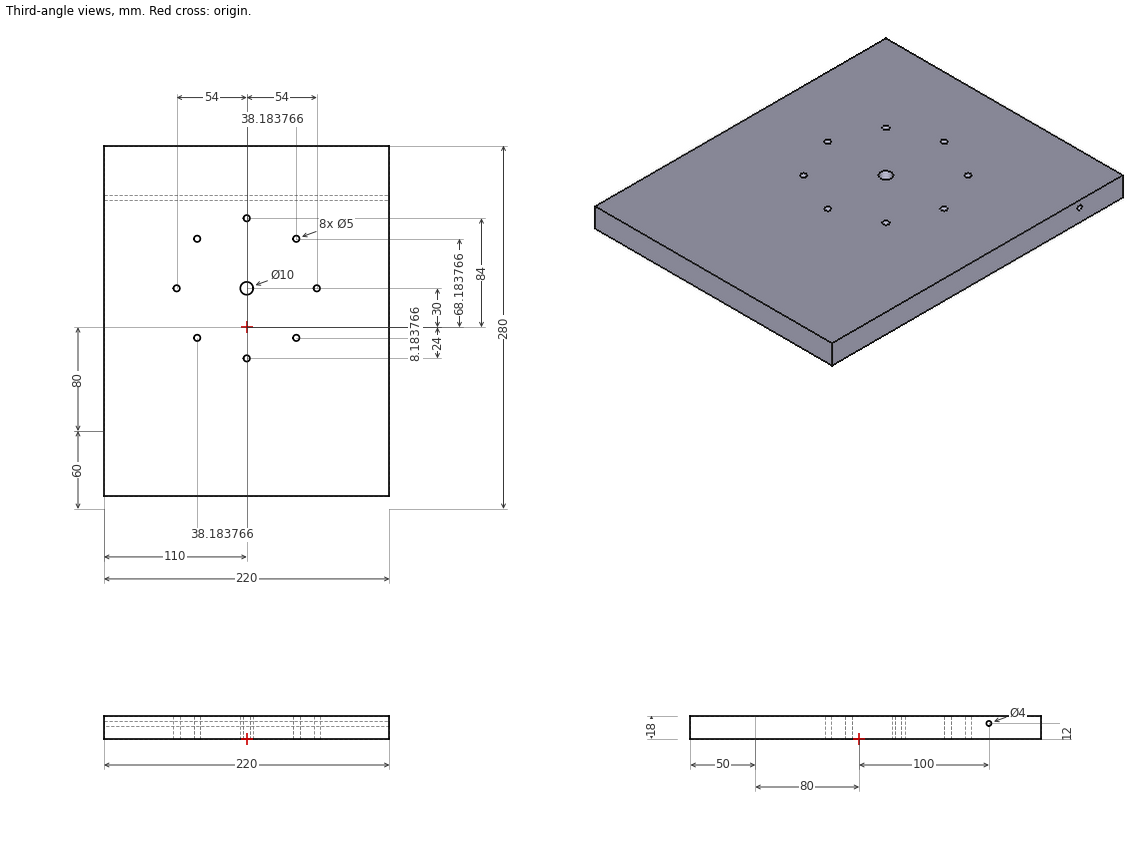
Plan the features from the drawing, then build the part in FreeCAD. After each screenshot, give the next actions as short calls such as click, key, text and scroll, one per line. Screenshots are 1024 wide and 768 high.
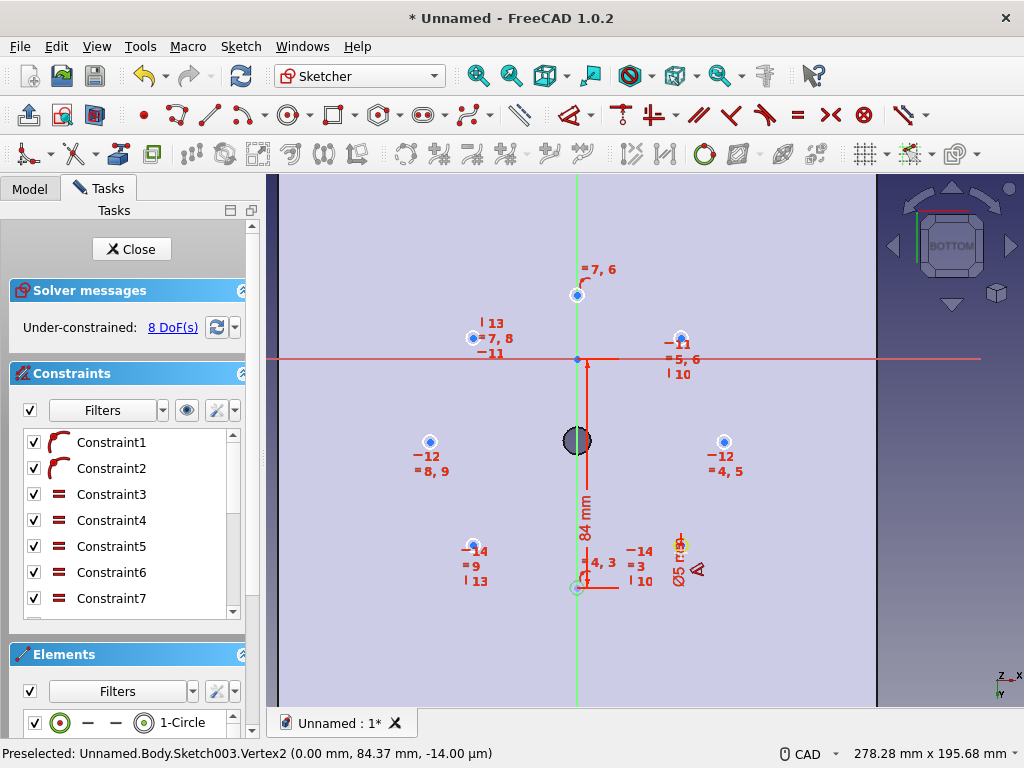
click(724, 442)
click(651, 325)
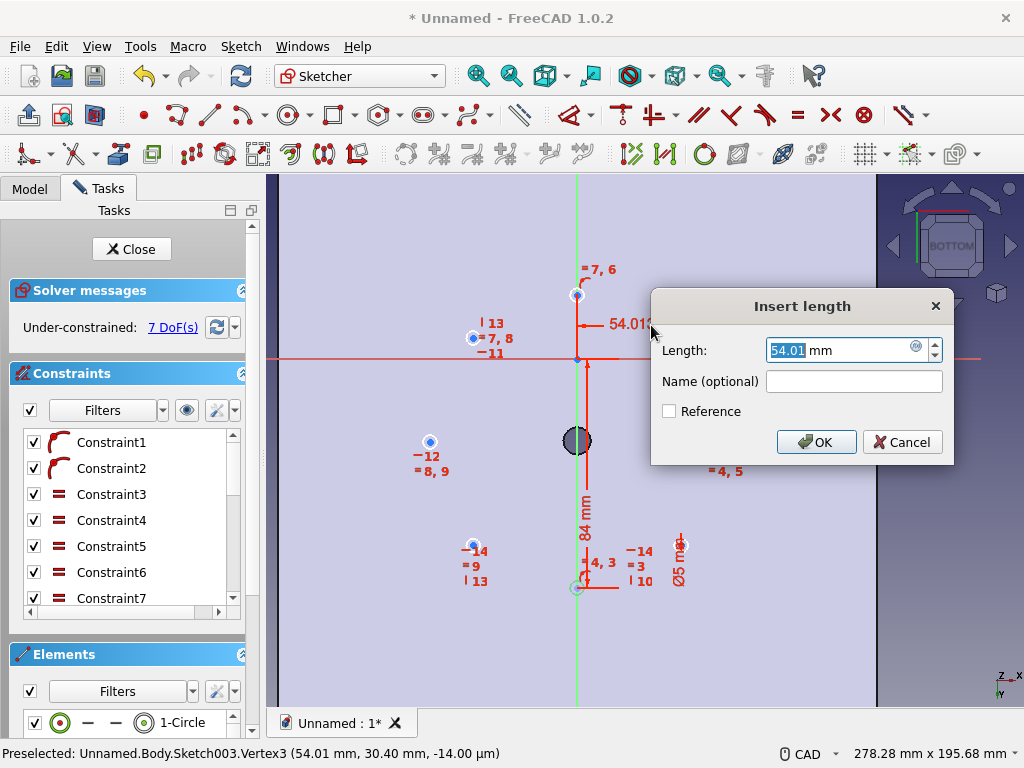
text(54)
key(Return)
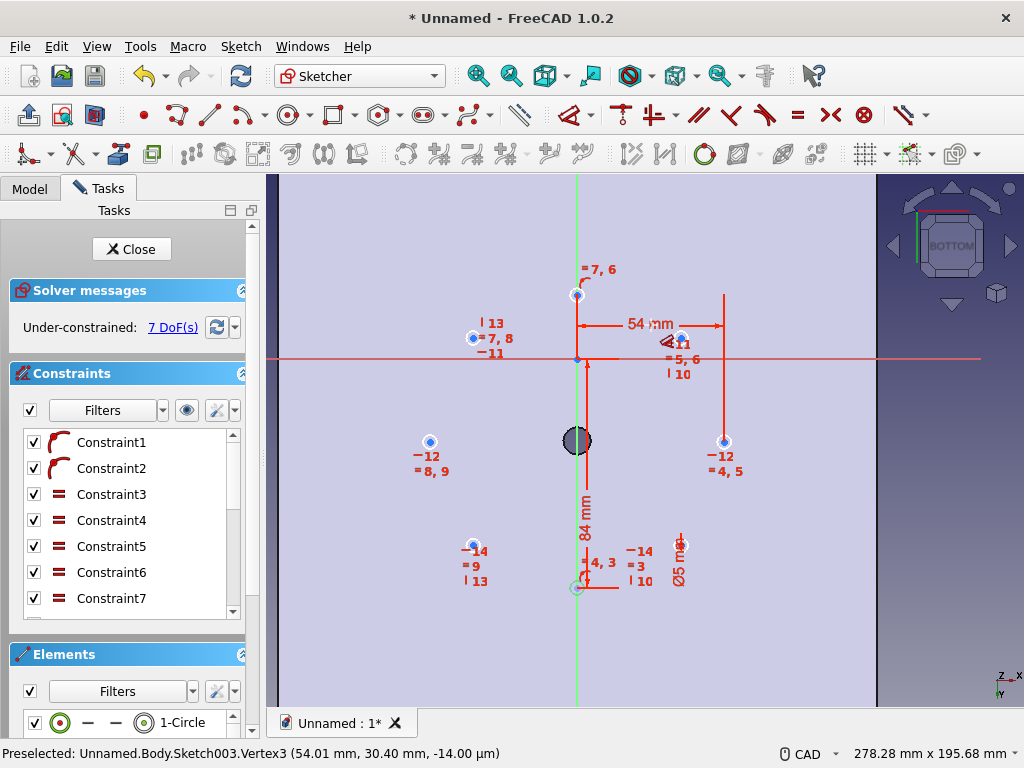
click(724, 442)
click(758, 401)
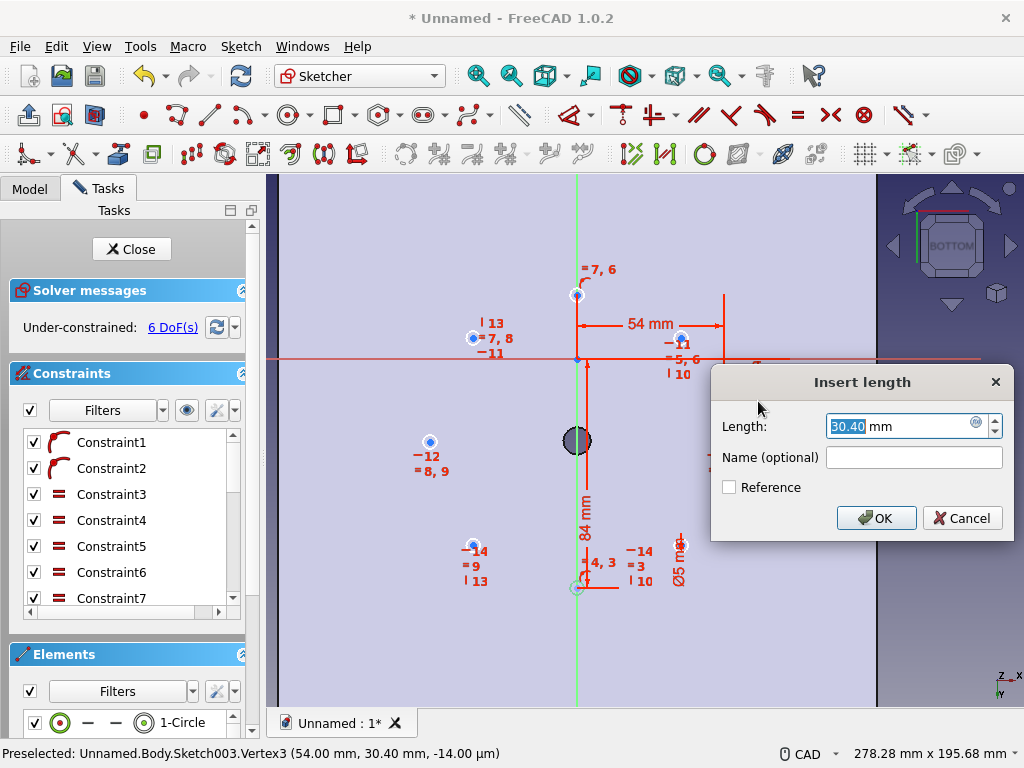
text(30)
key(Return)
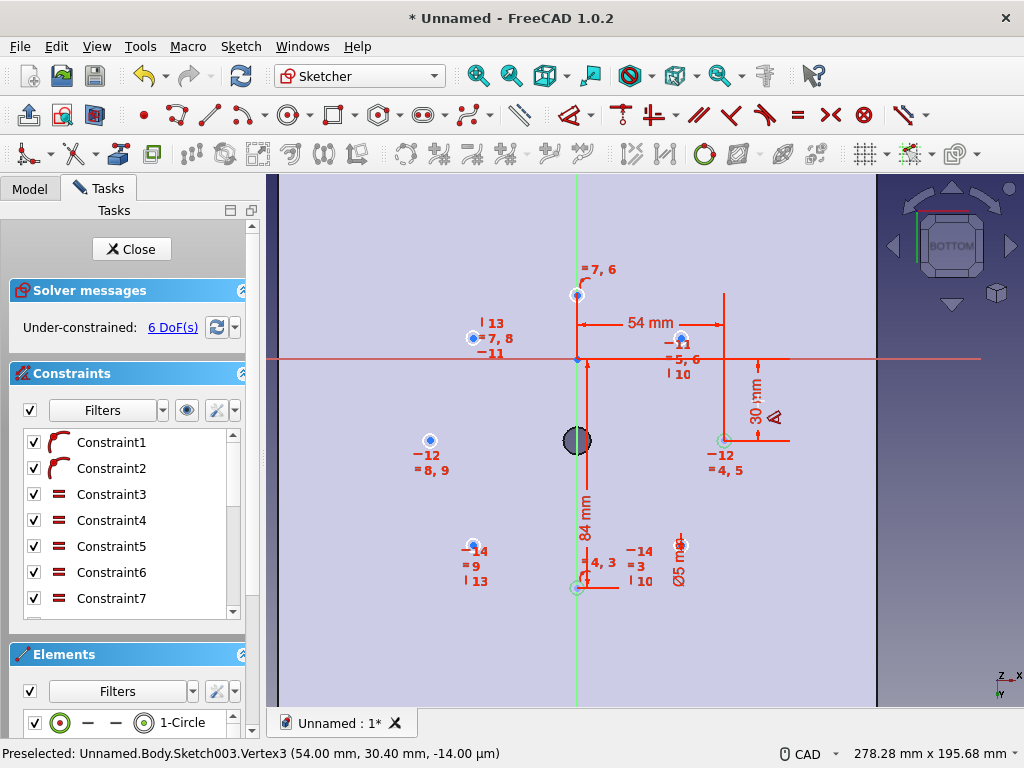
click(577, 295)
click(611, 305)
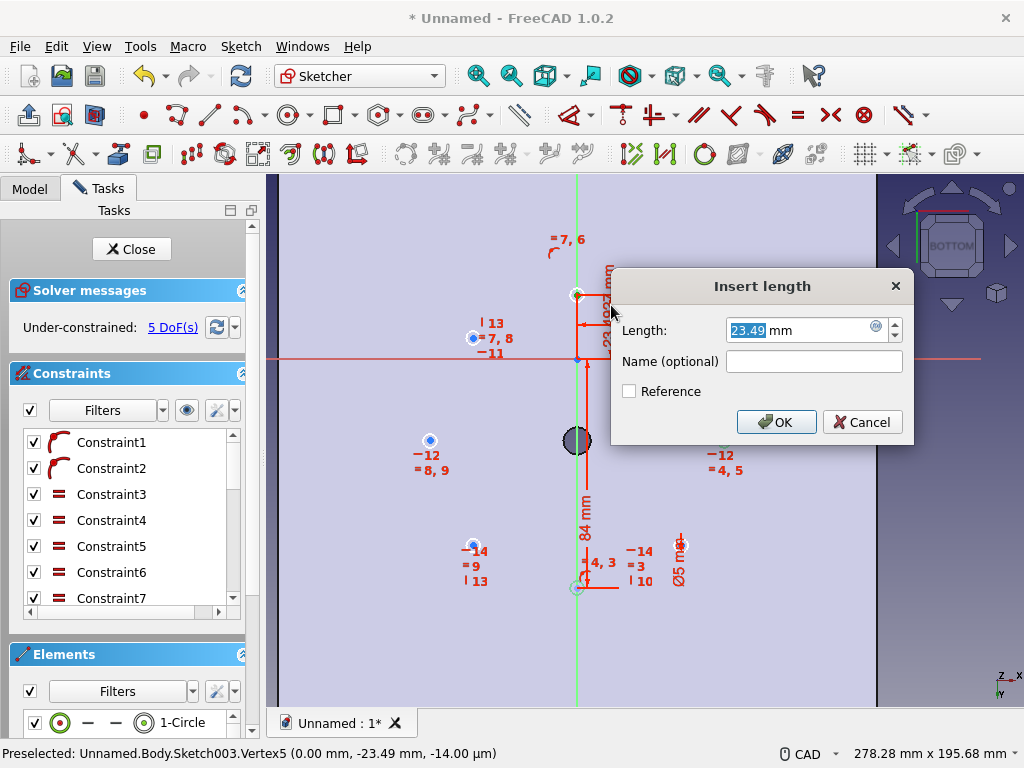
text(24)
key(Return)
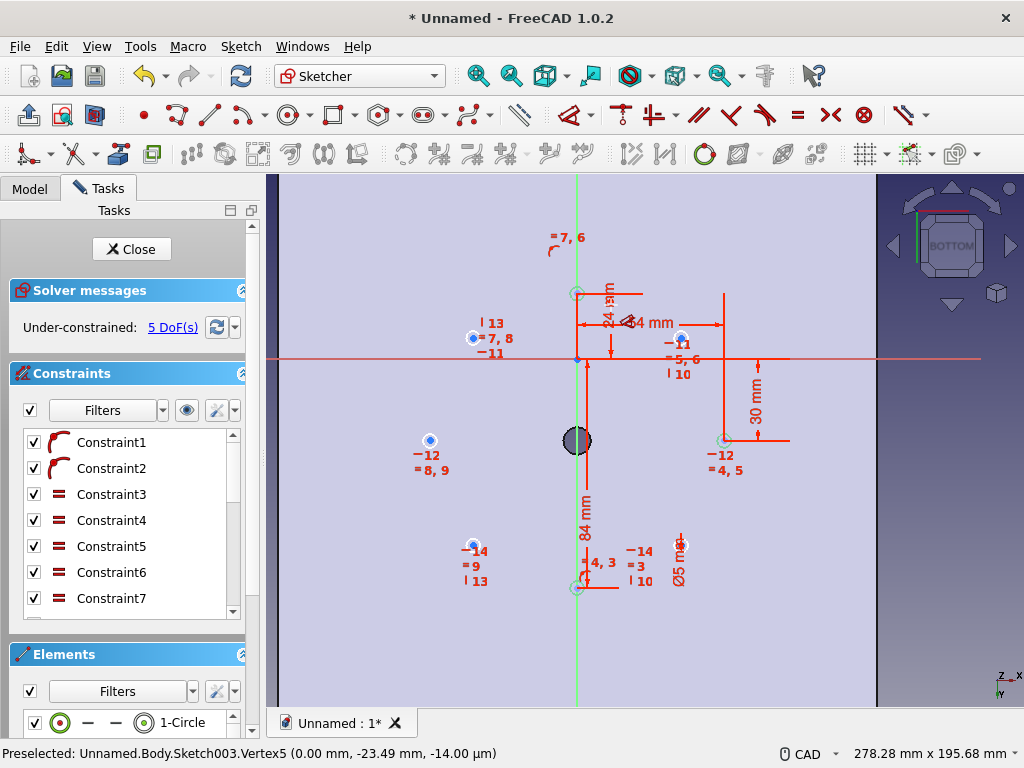
click(430, 441)
click(504, 325)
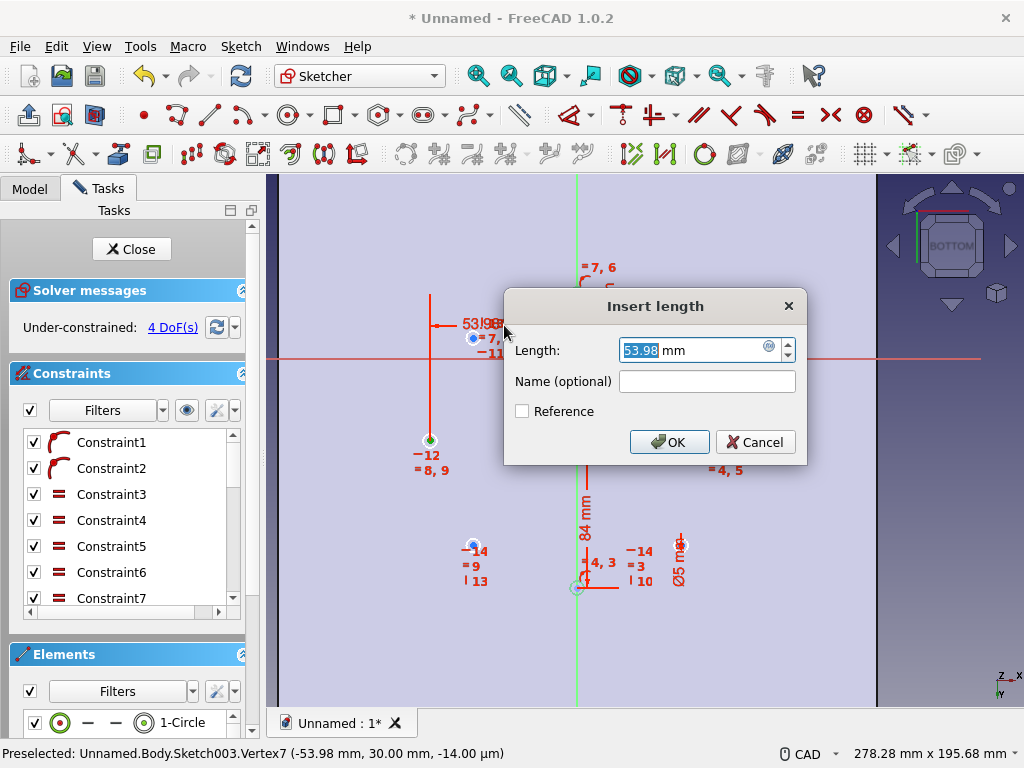
text(54)
key(Return)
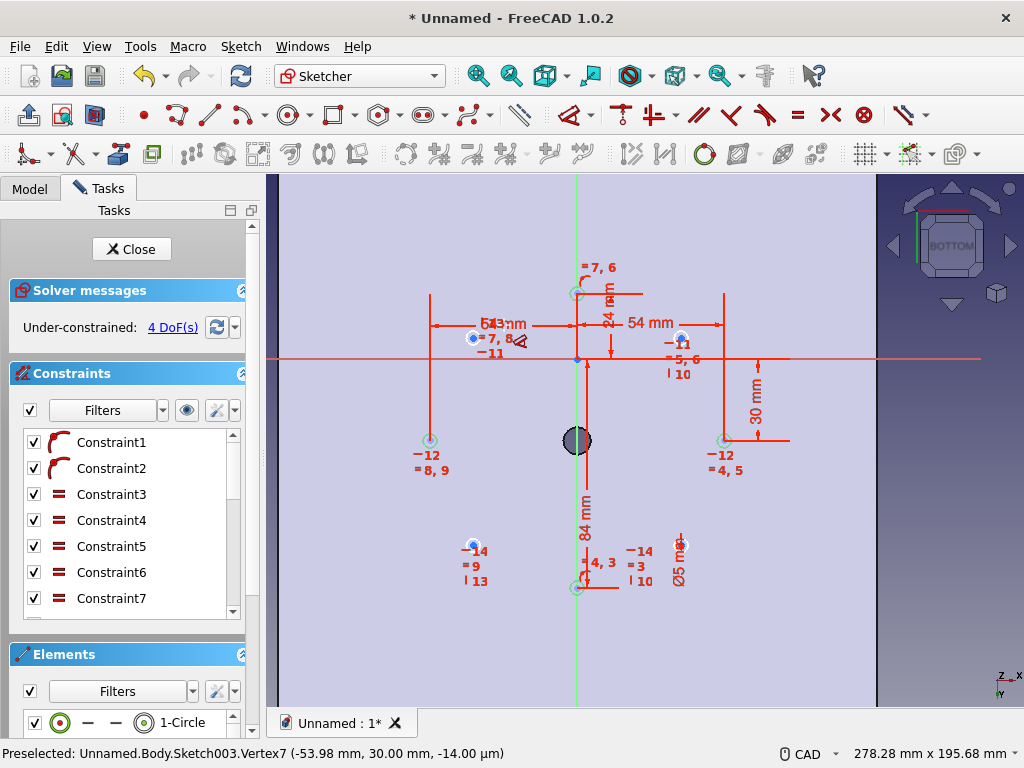
scroll(681, 338, up, 3)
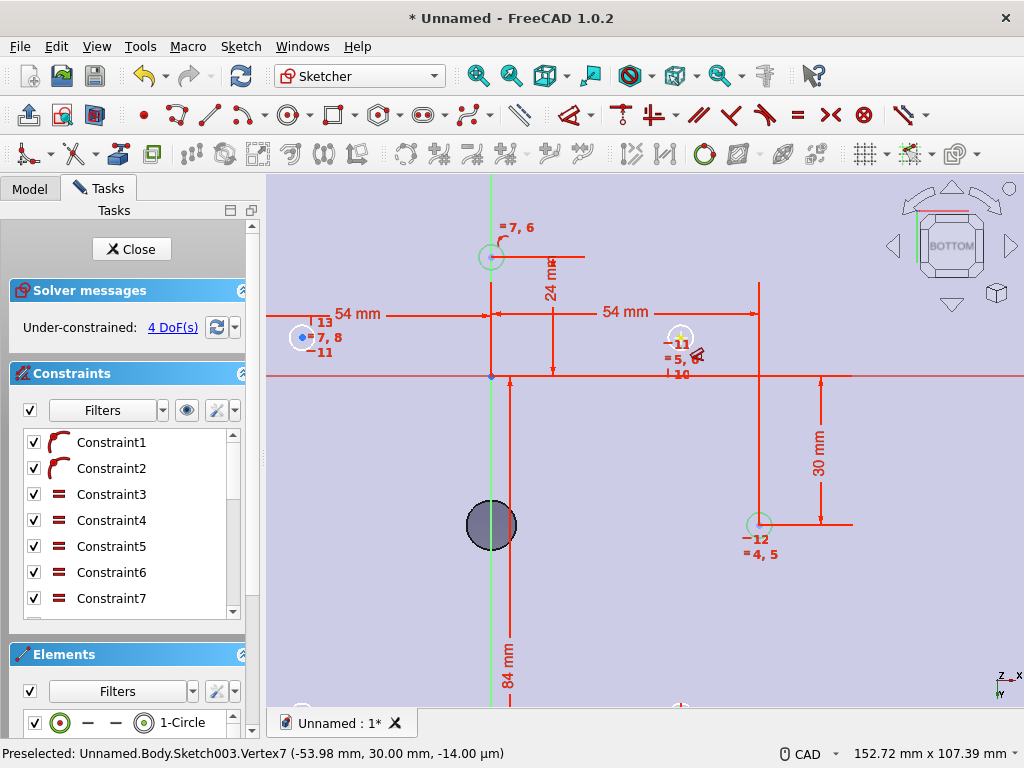
click(681, 338)
click(715, 357)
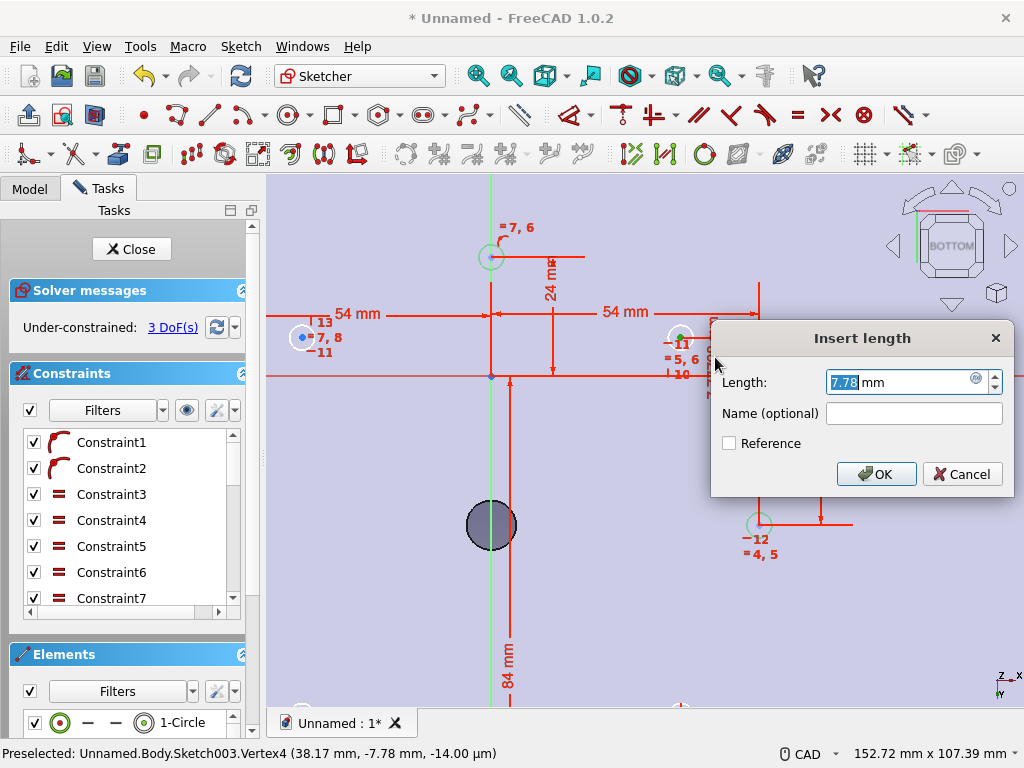
text(8.183766)
key(Return)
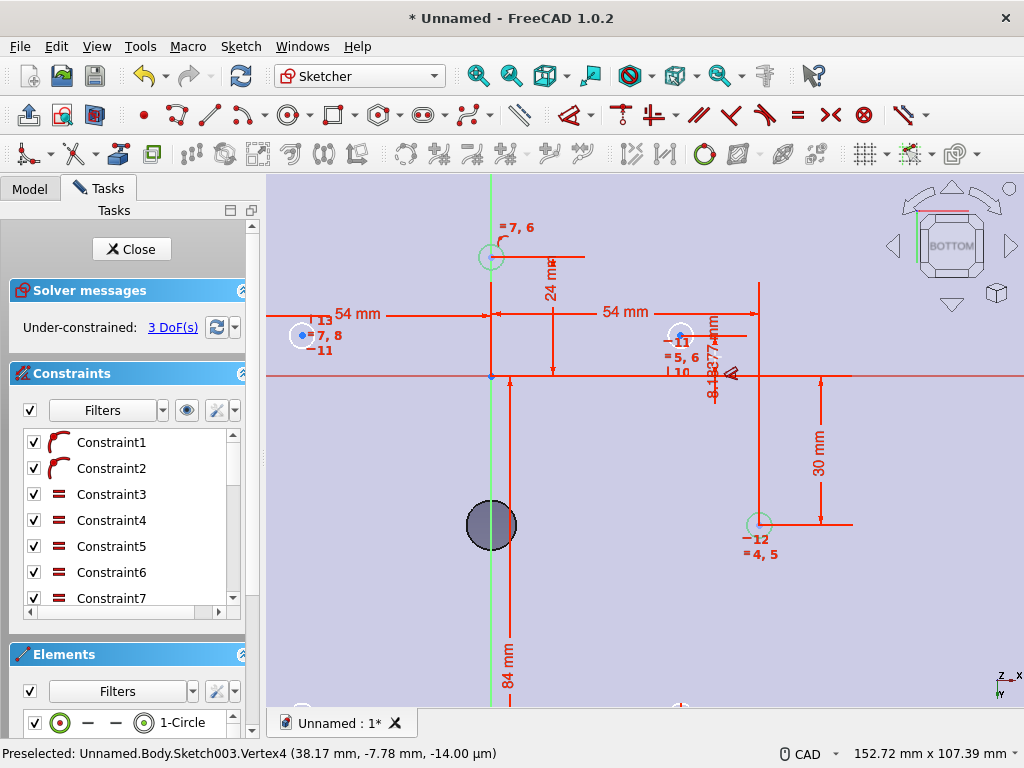
scroll(680, 337, down, 3)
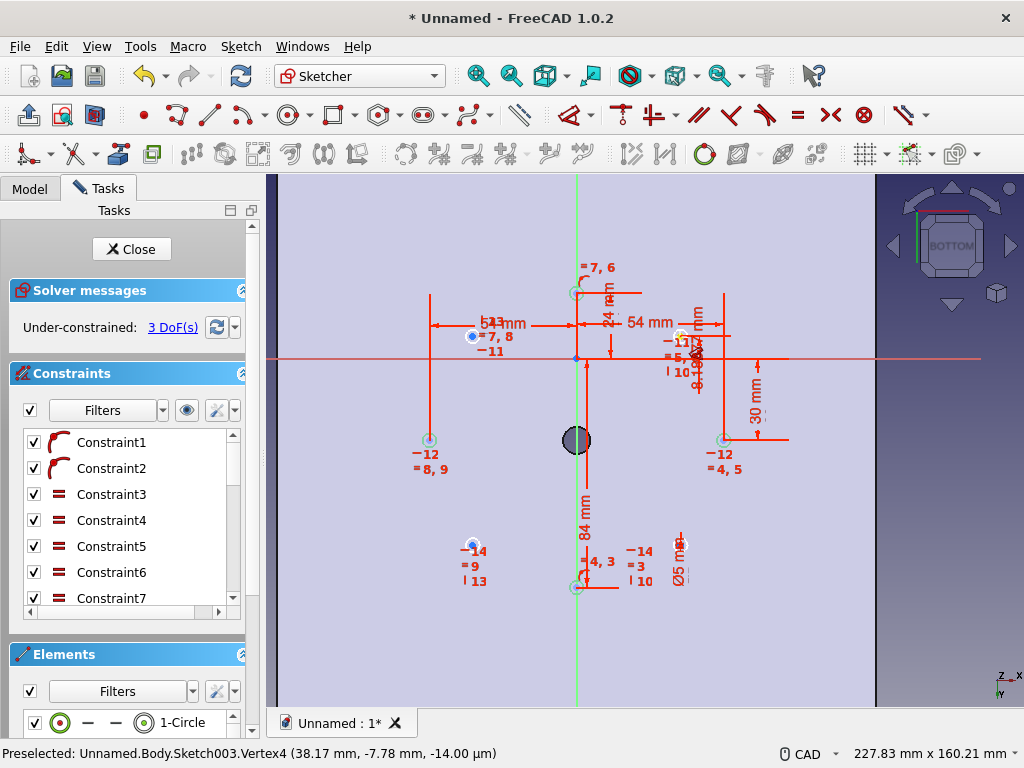
click(681, 545)
click(605, 579)